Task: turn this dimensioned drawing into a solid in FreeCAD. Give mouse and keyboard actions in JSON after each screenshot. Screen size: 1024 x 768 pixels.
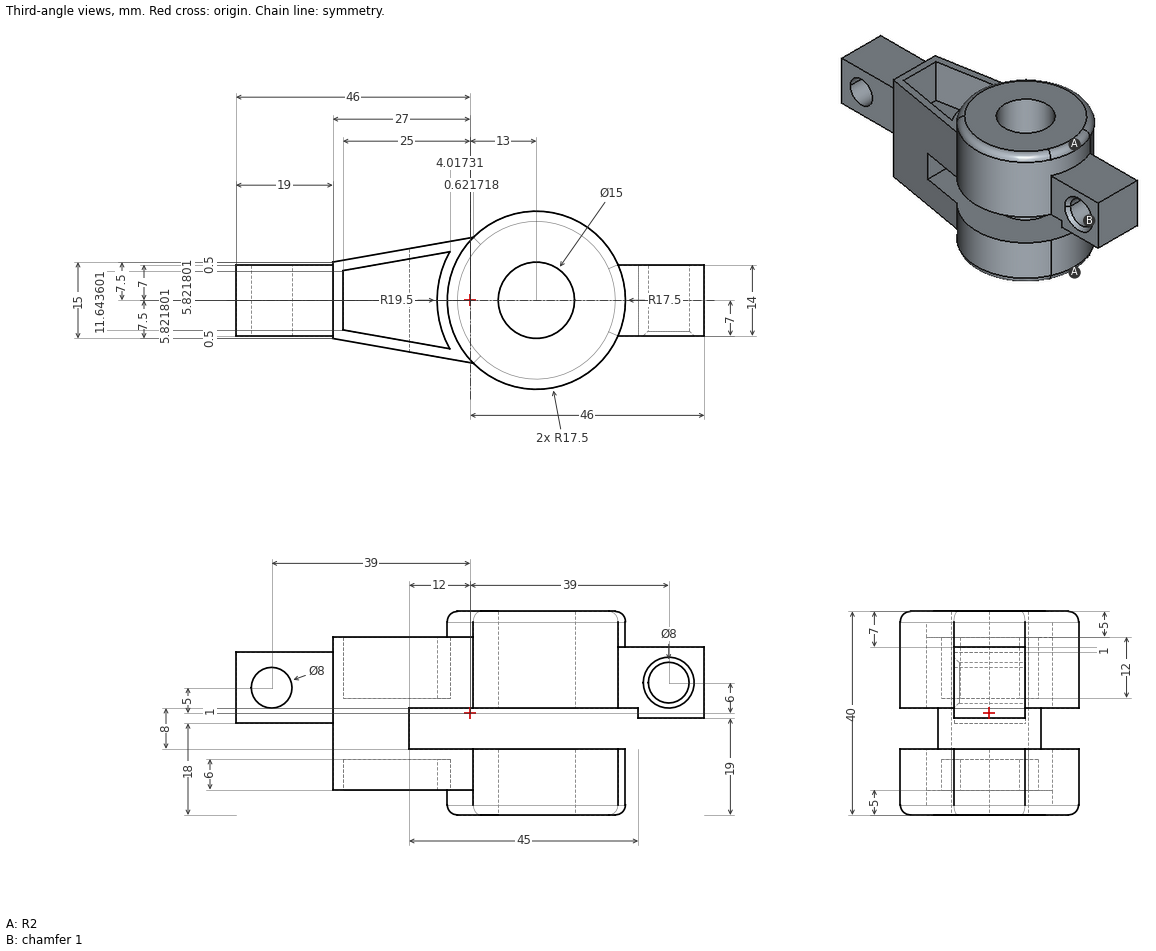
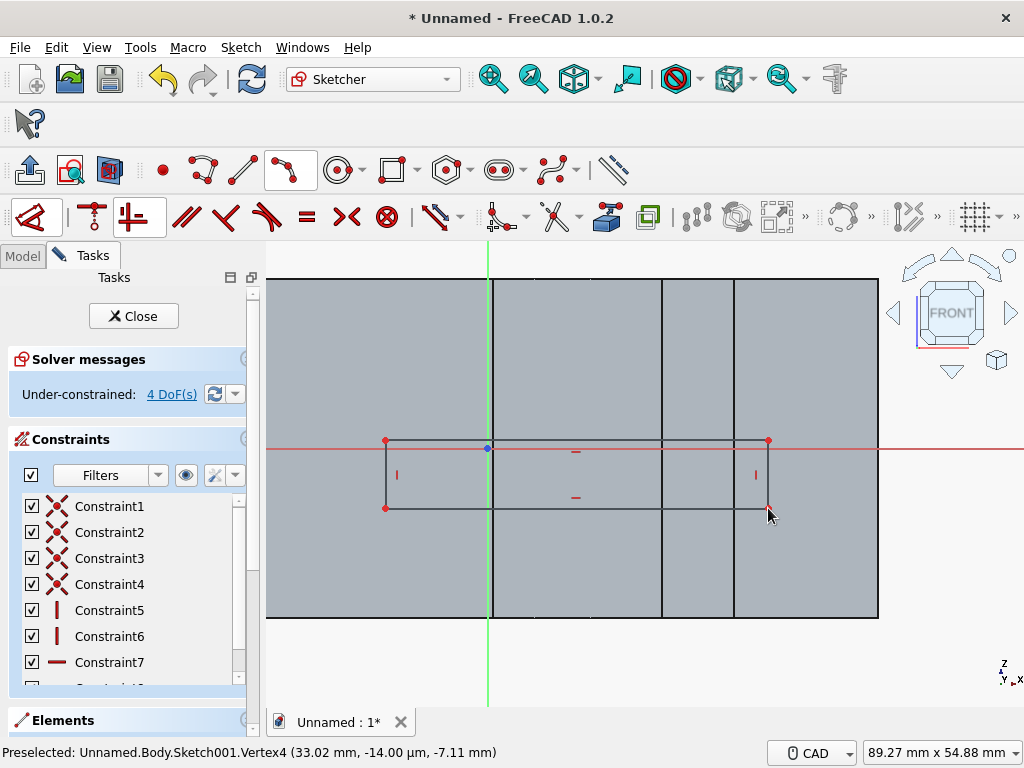
{"action": "left_click", "coordinate": [386, 461]}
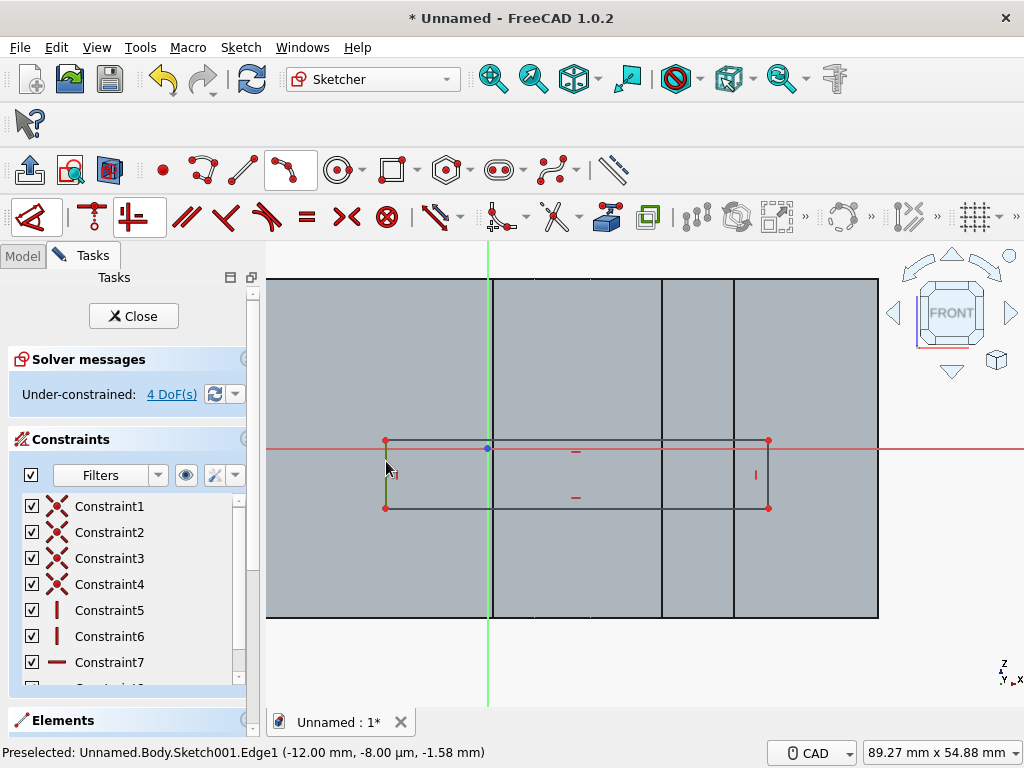
{"action": "left_click", "coordinate": [56, 218]}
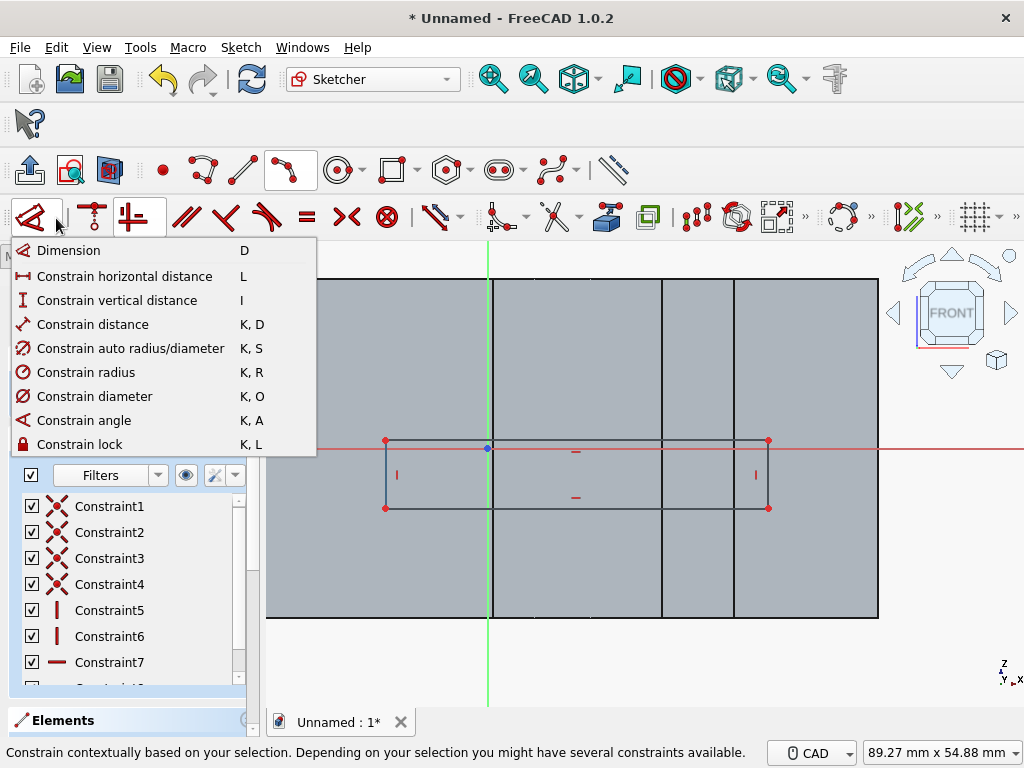
{"action": "left_click", "coordinate": [164, 300]}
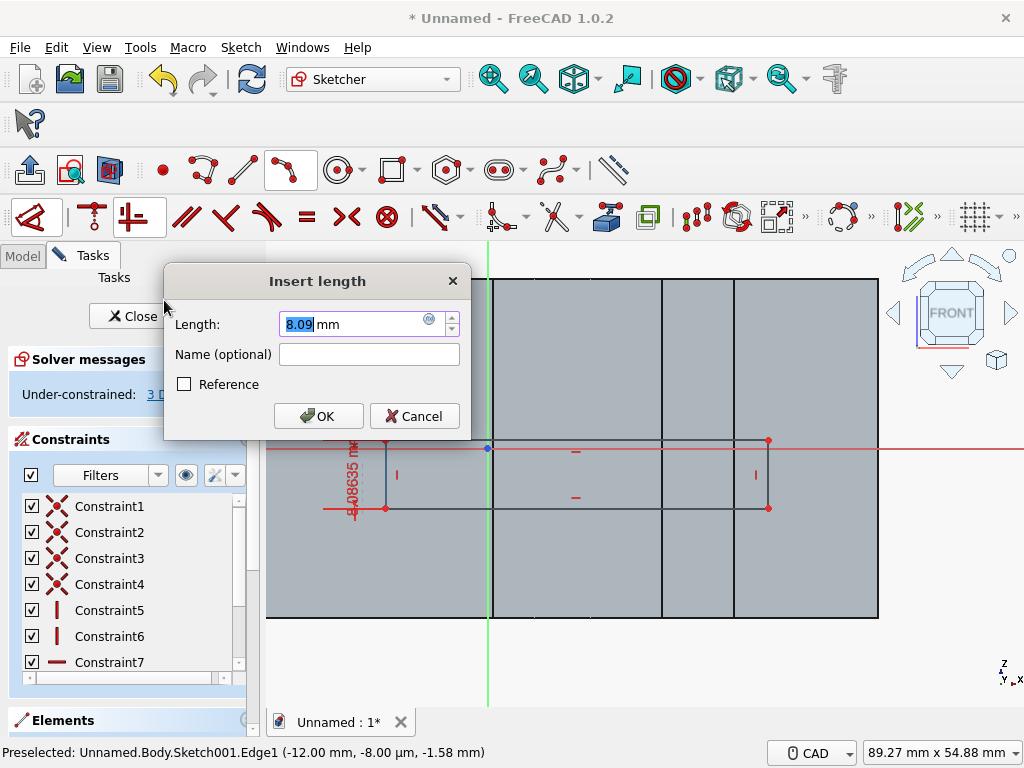
{"action": "type", "text": "8"}
{"action": "key", "text": "Return"}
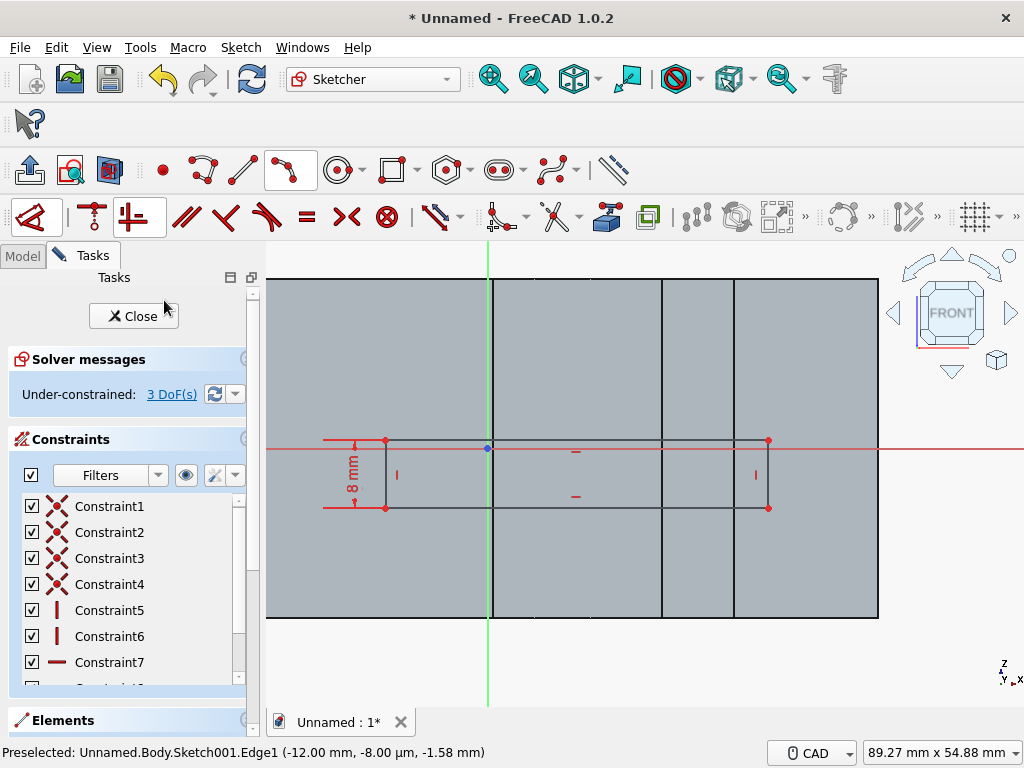
{"action": "left_click", "coordinate": [500, 508]}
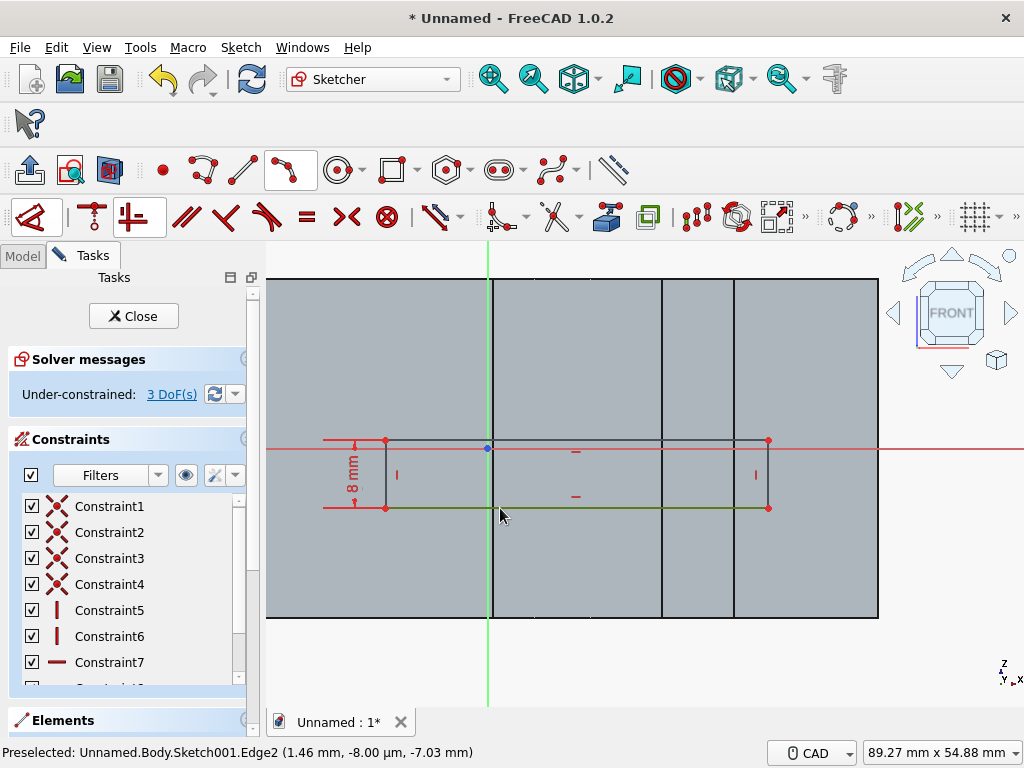
{"action": "key", "text": "l"}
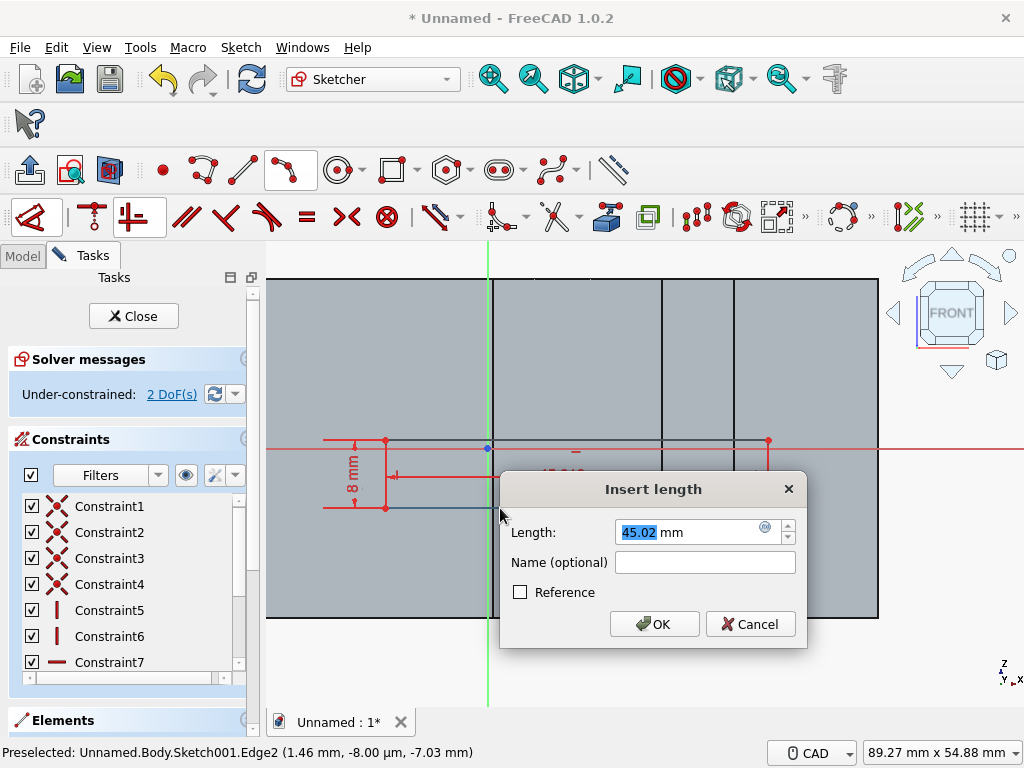
{"action": "type", "text": "45"}
{"action": "key", "text": "Return"}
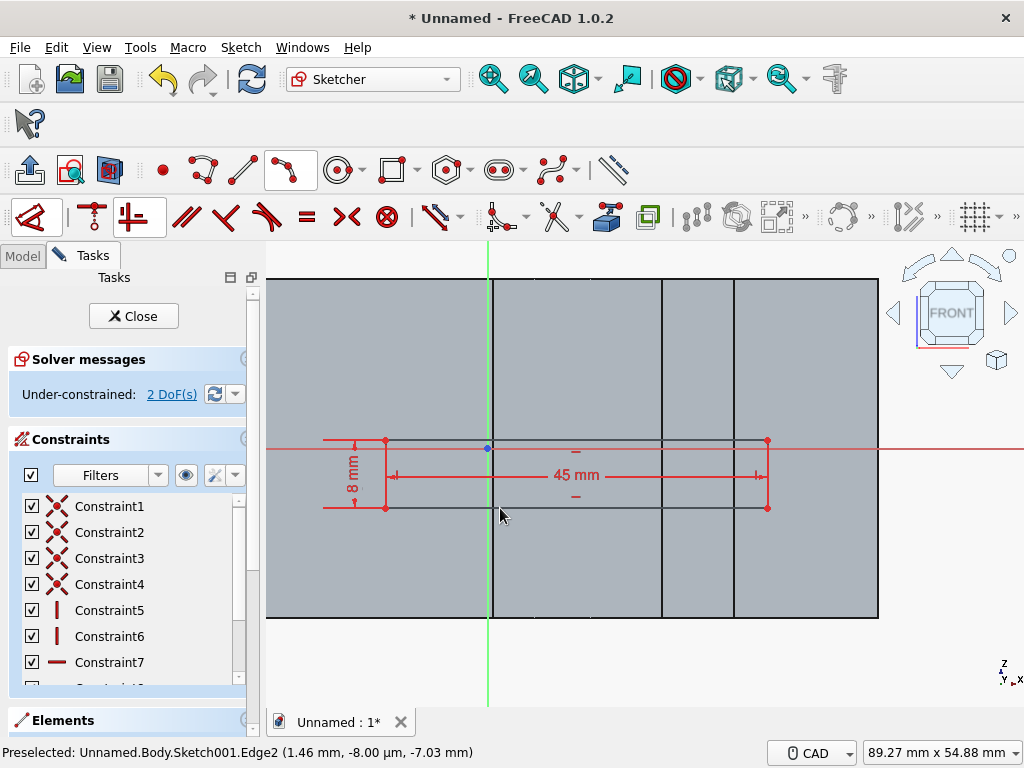
{"action": "scroll", "coordinate": [386, 440], "scroll_direction": "up", "scroll_amount": 8}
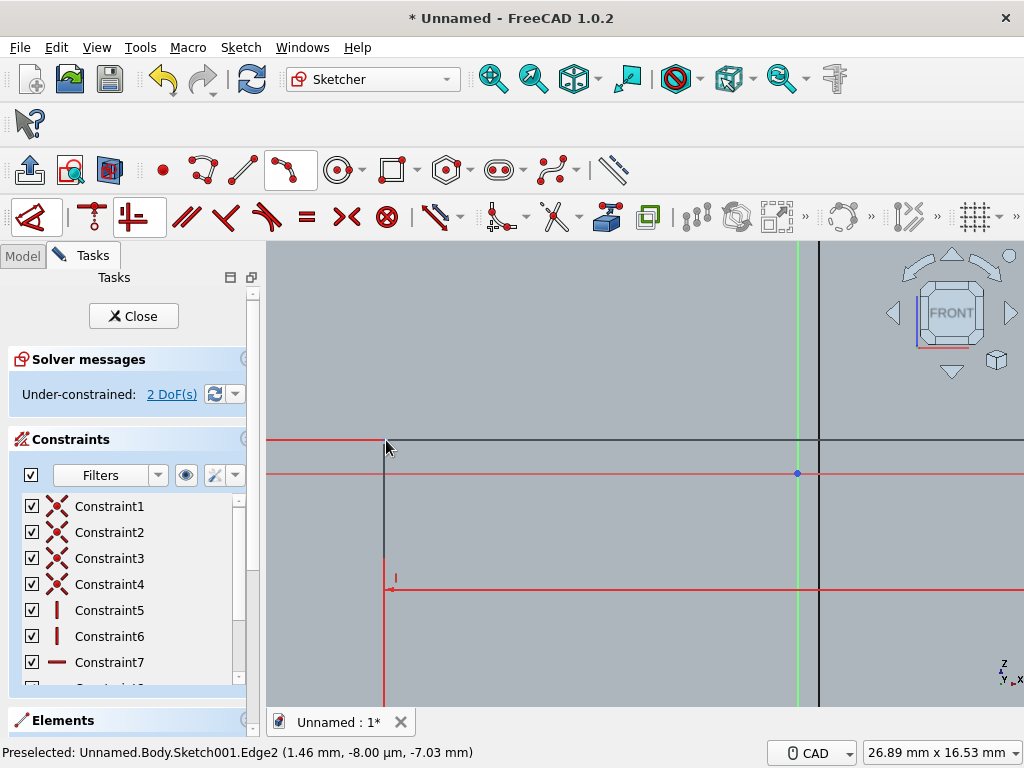
{"action": "left_click", "coordinate": [384, 440]}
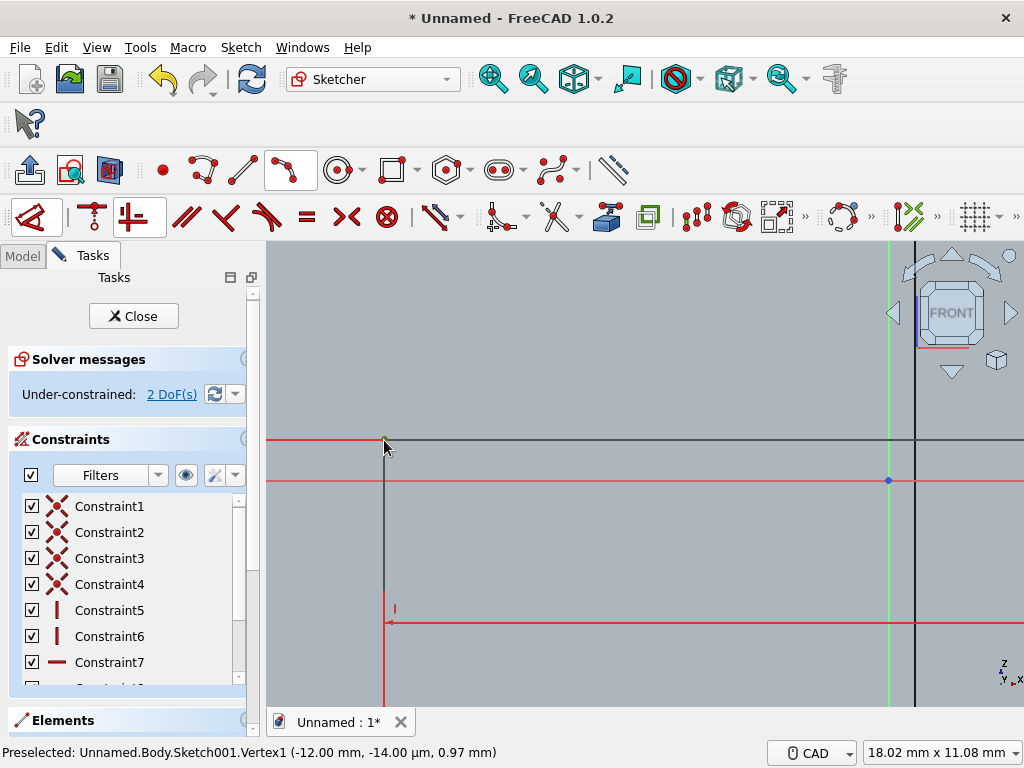
{"action": "left_click", "coordinate": [56, 218]}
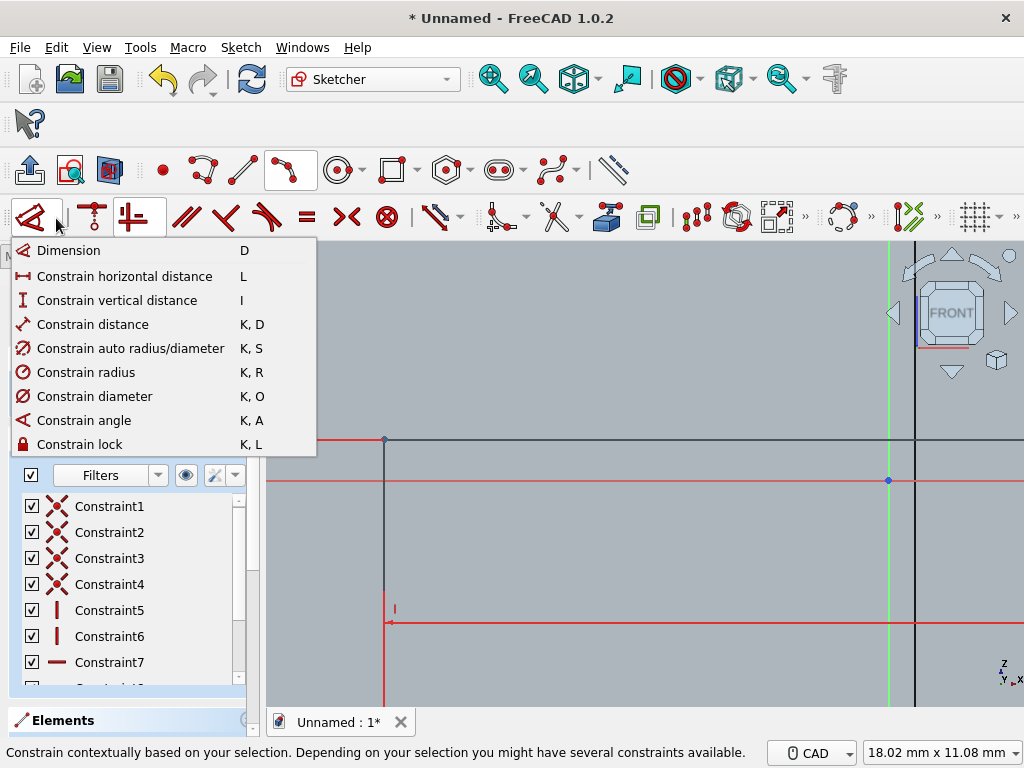
{"action": "left_click", "coordinate": [164, 300]}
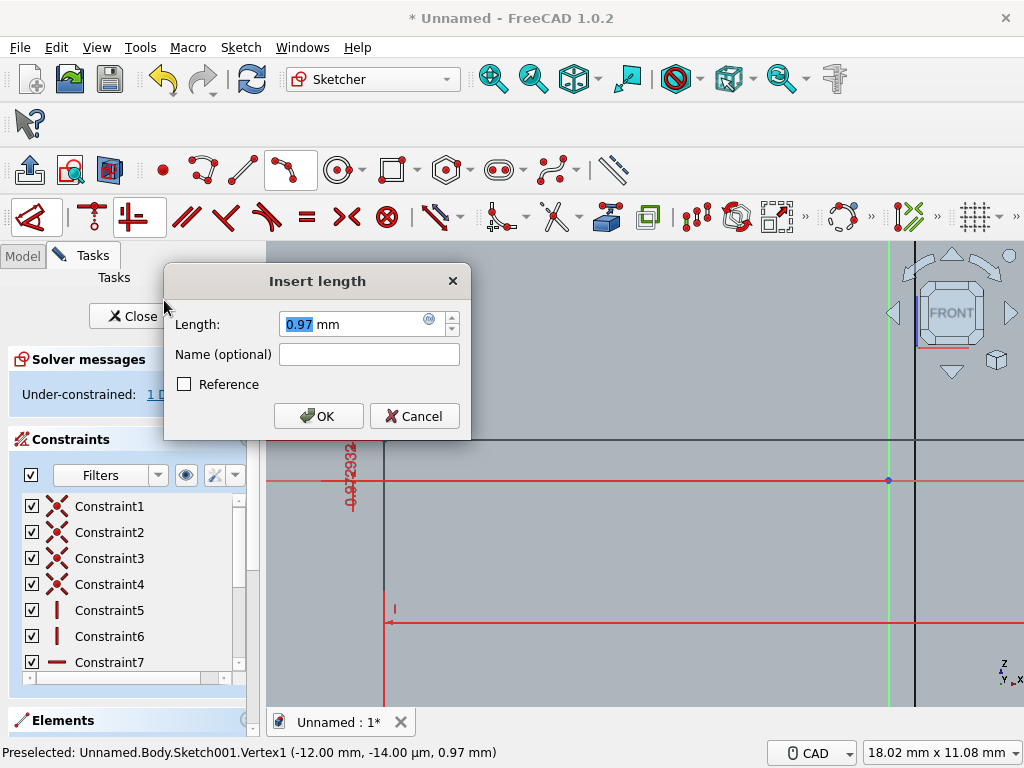
{"action": "type", "text": "1"}
{"action": "key", "text": "Return"}